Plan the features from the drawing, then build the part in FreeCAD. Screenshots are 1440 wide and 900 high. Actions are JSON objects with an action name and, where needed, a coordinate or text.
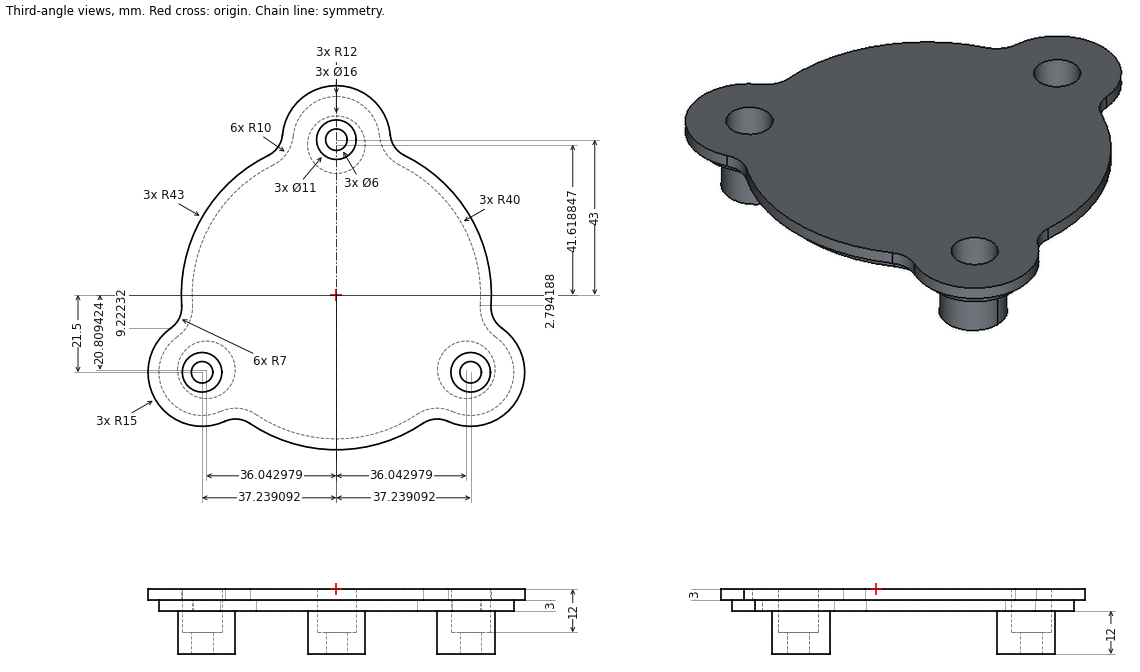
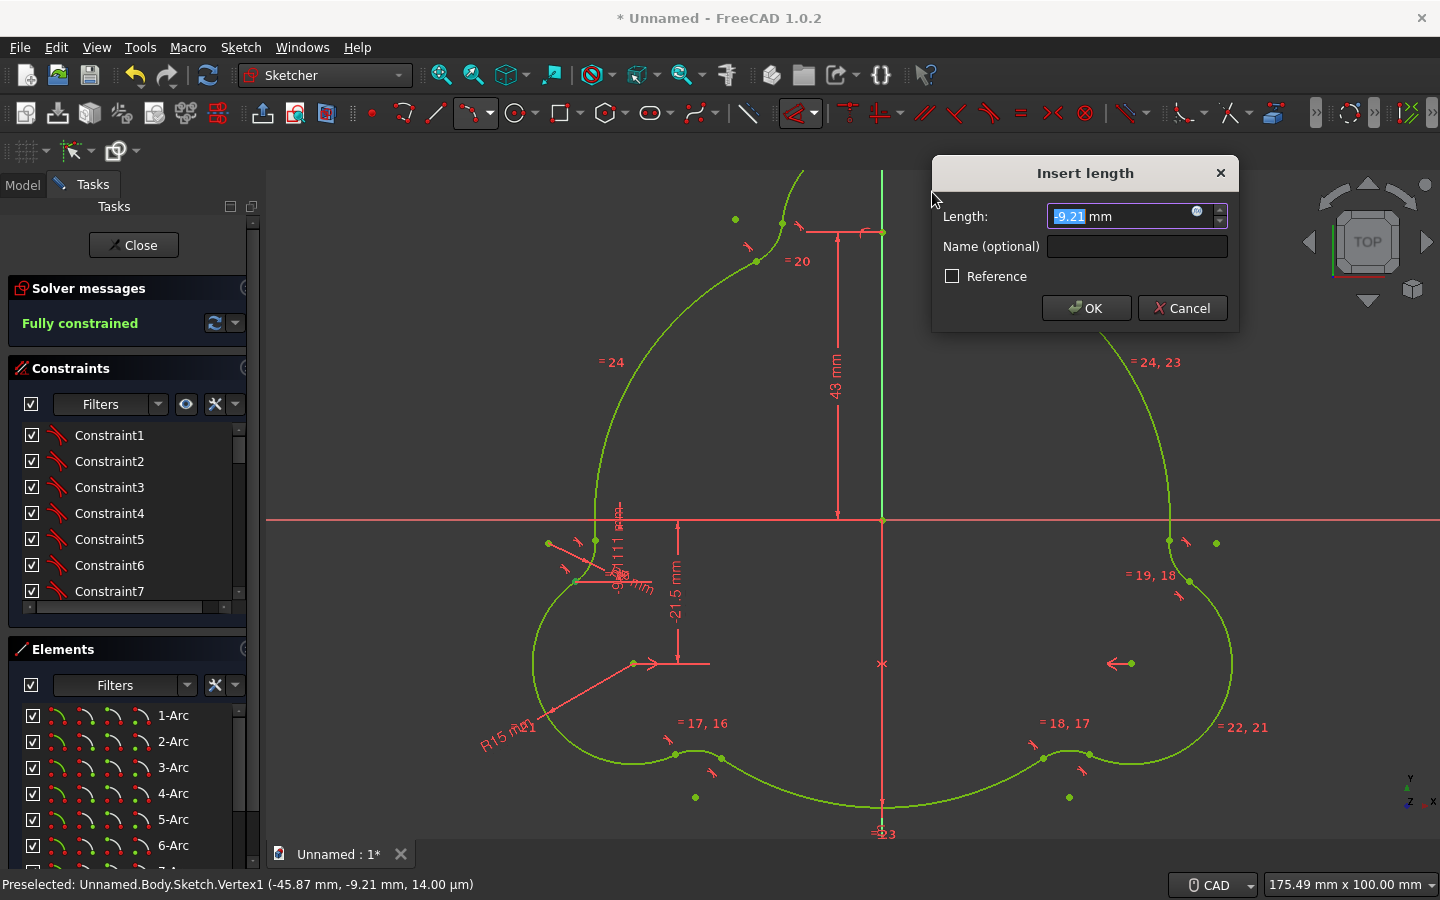
{"action": "type", "text": "-9.22232"}
{"action": "key", "text": "Return"}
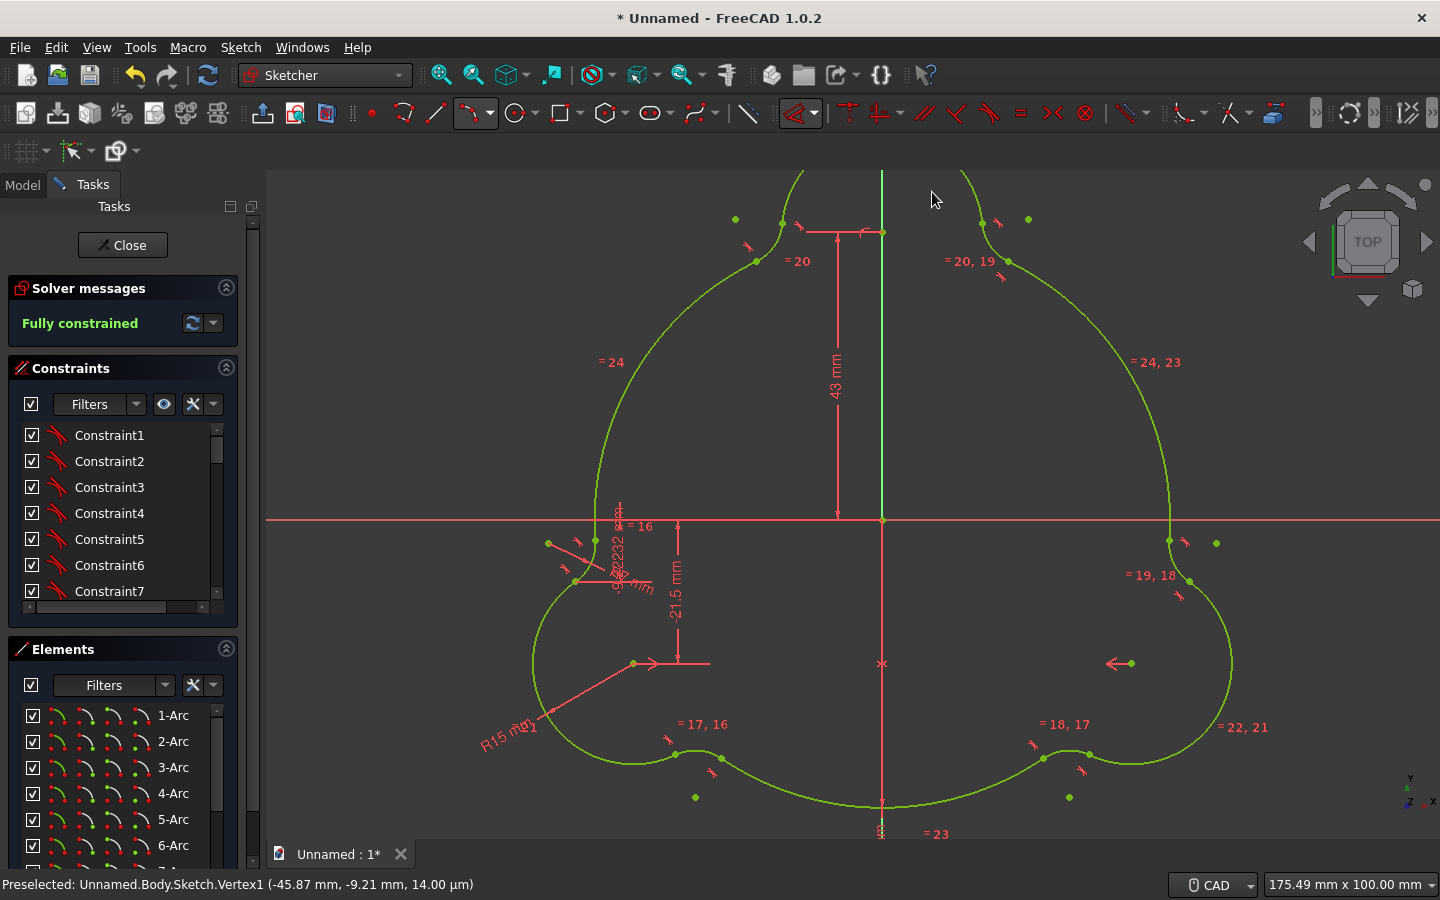
{"action": "left_click", "coordinate": [123, 245]}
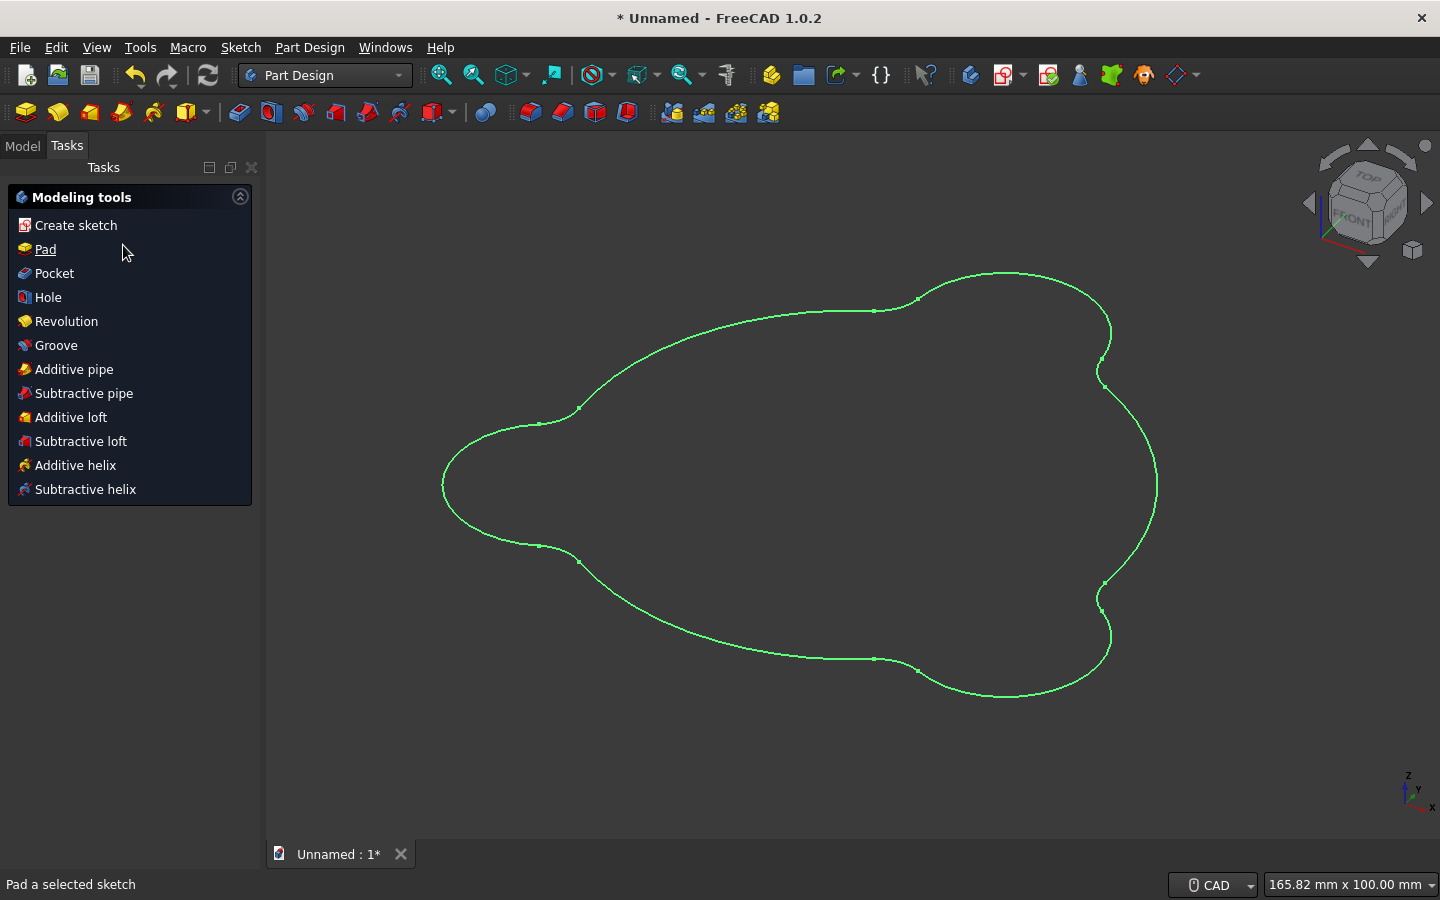
{"action": "left_click", "coordinate": [26, 112]}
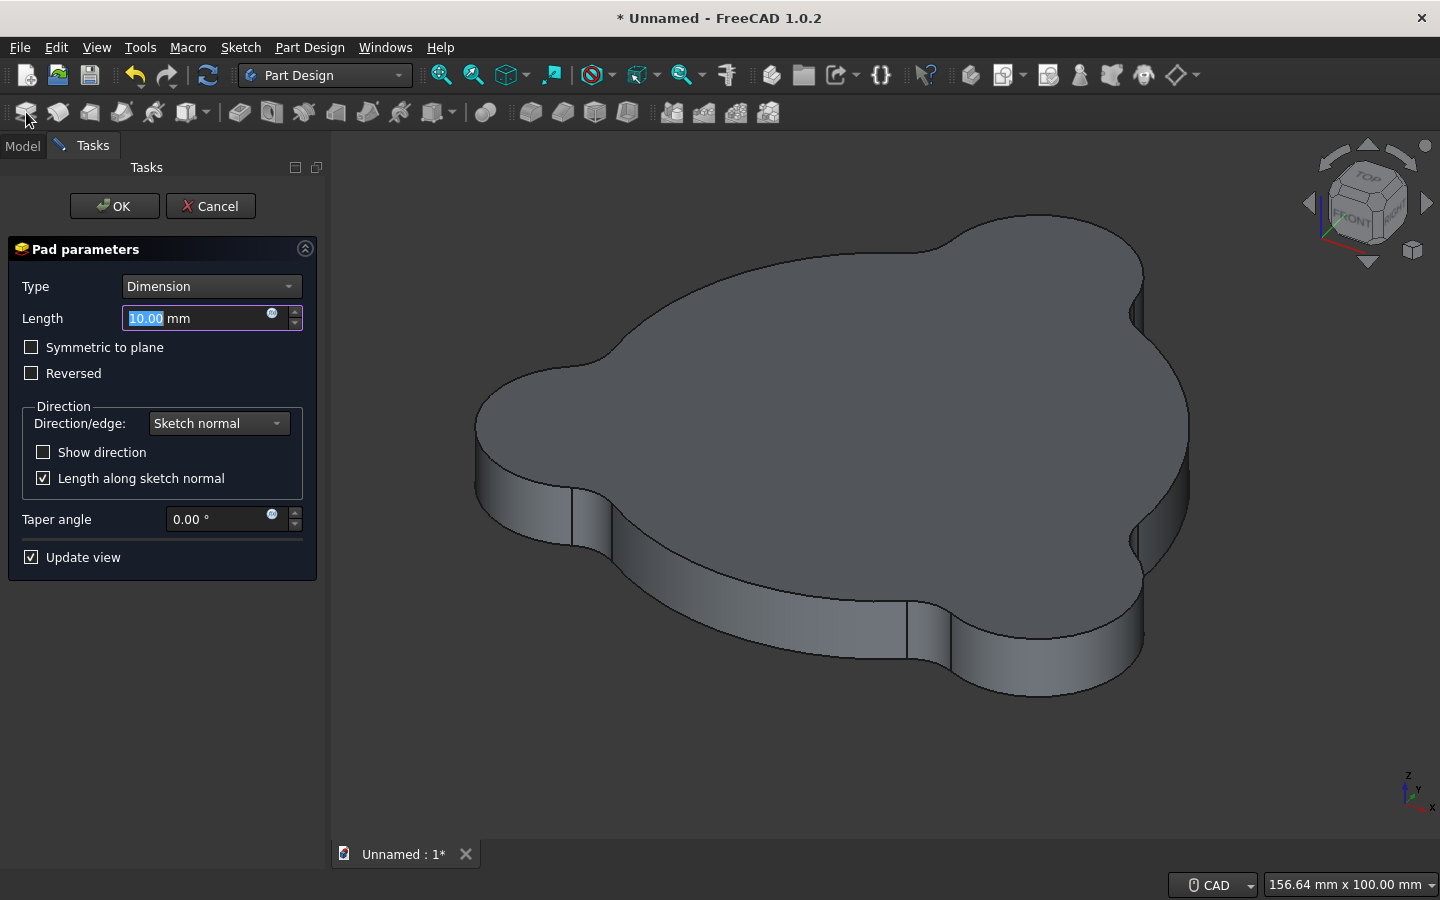
{"action": "type", "text": "3"}
{"action": "key", "text": "Tab"}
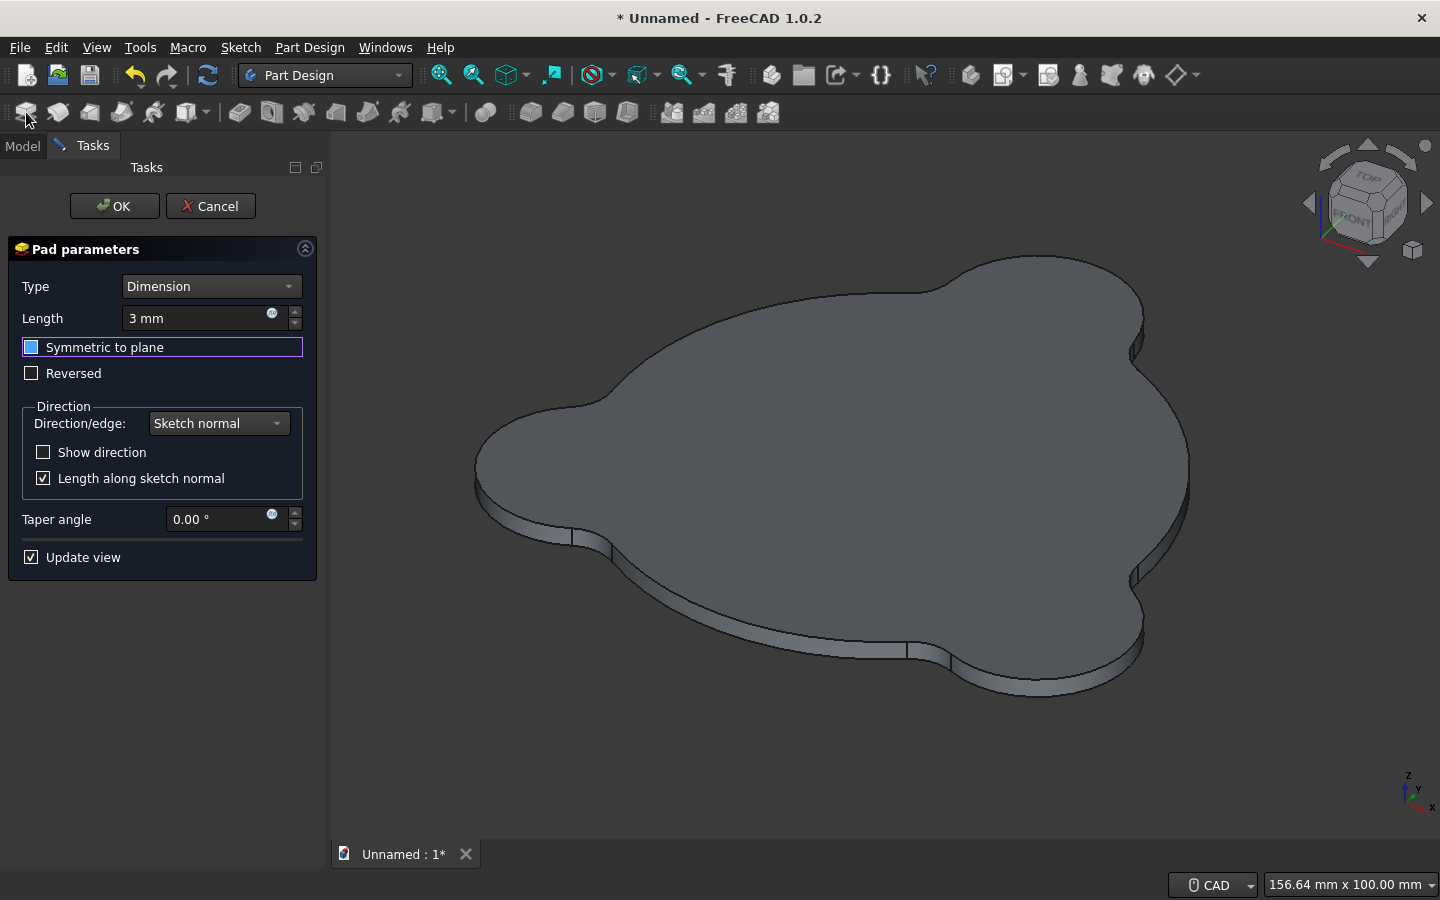
{"action": "left_click", "coordinate": [30, 373]}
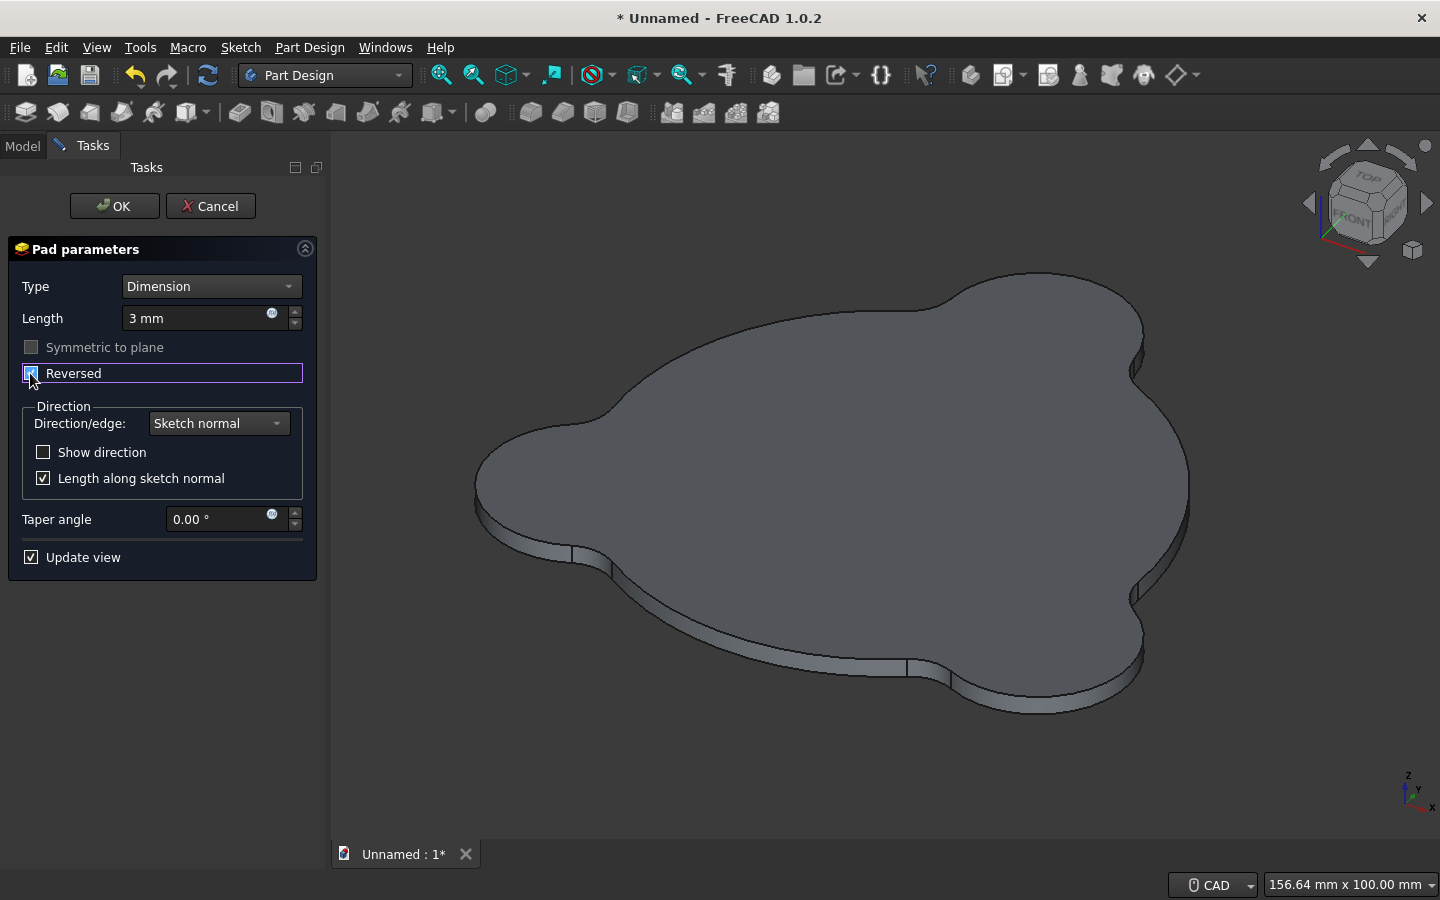
{"action": "left_click", "coordinate": [115, 206]}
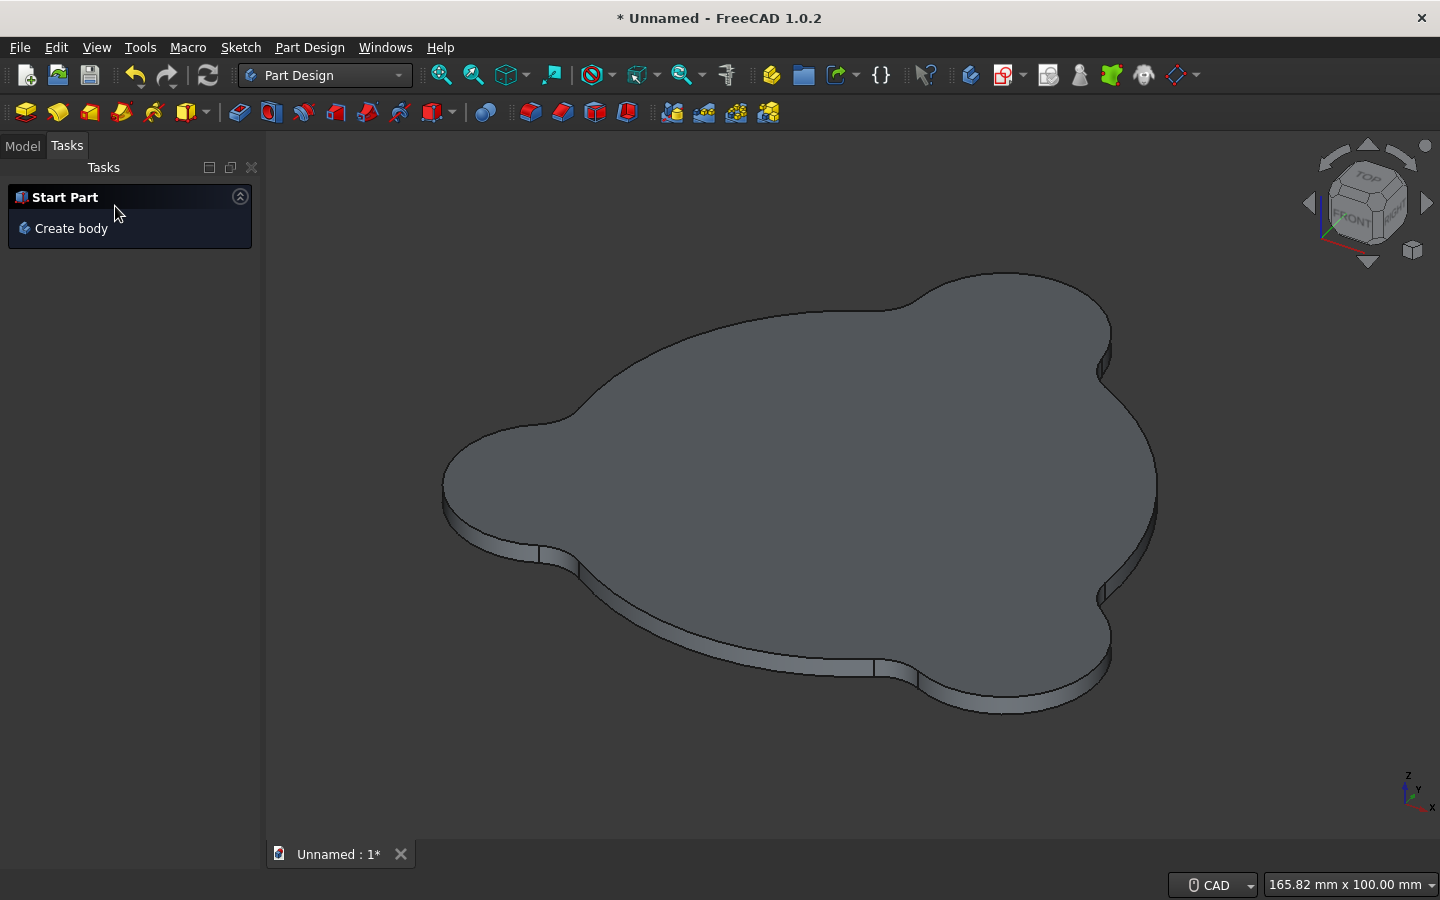
{"action": "key", "text": "5"}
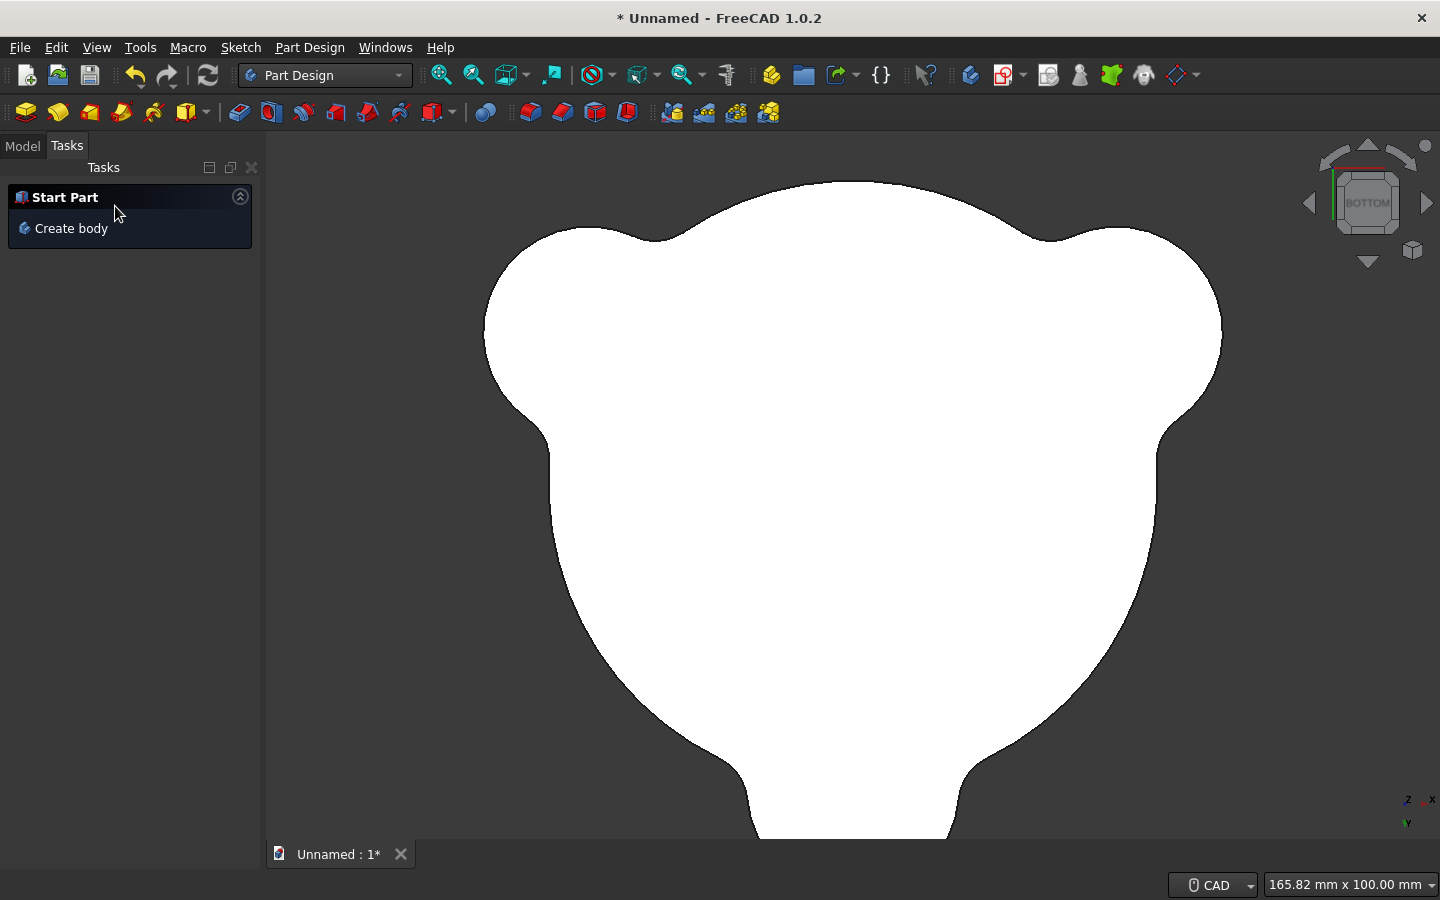
{"action": "left_click", "coordinate": [442, 76]}